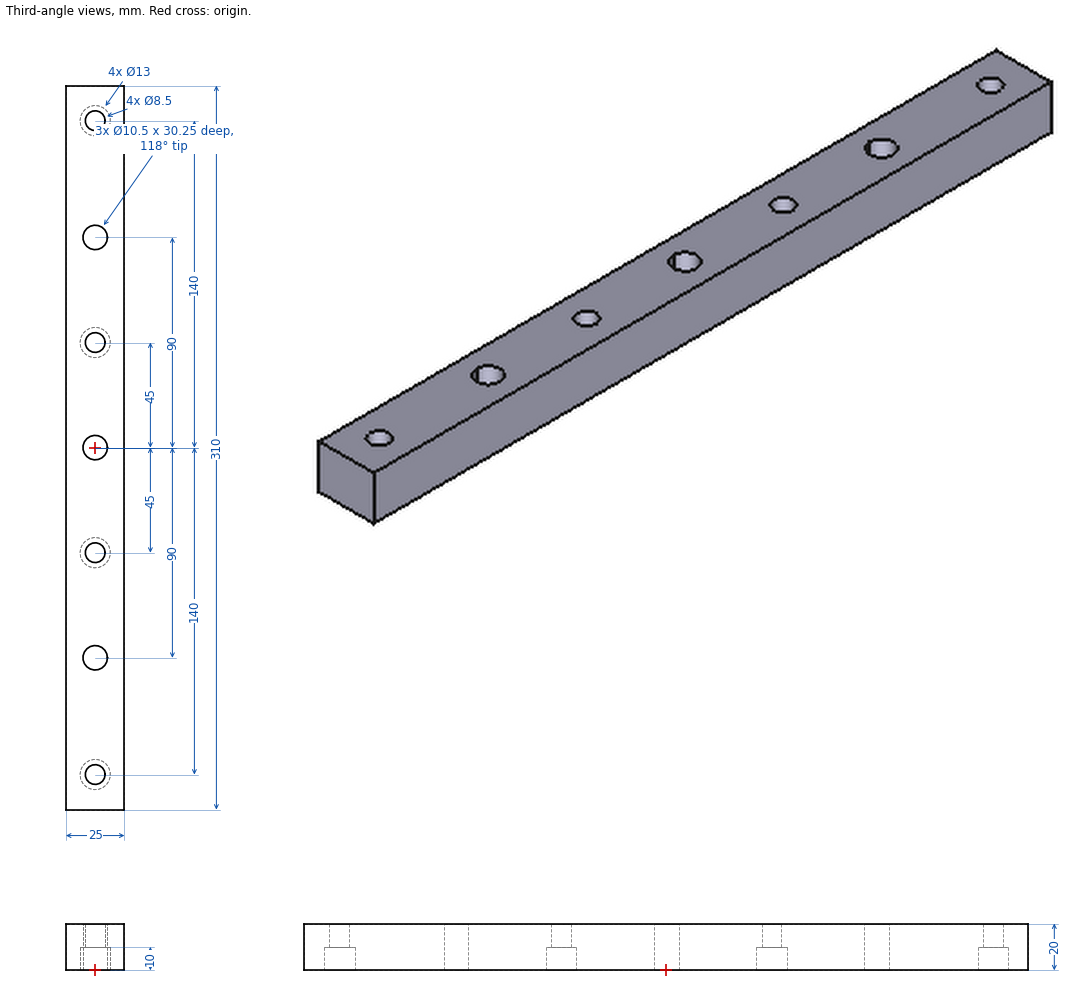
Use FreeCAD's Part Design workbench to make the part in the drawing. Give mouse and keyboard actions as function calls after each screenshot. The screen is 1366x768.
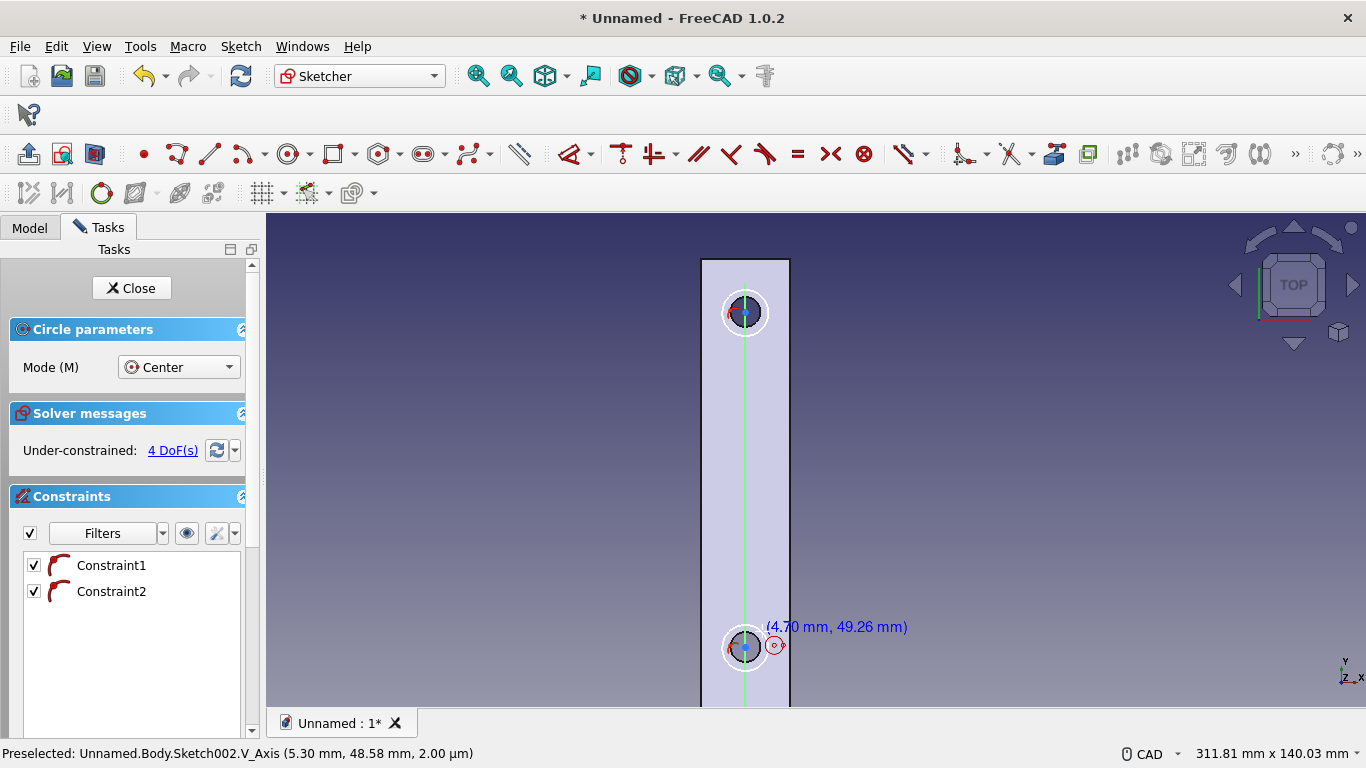
scroll(748, 311, down, 6)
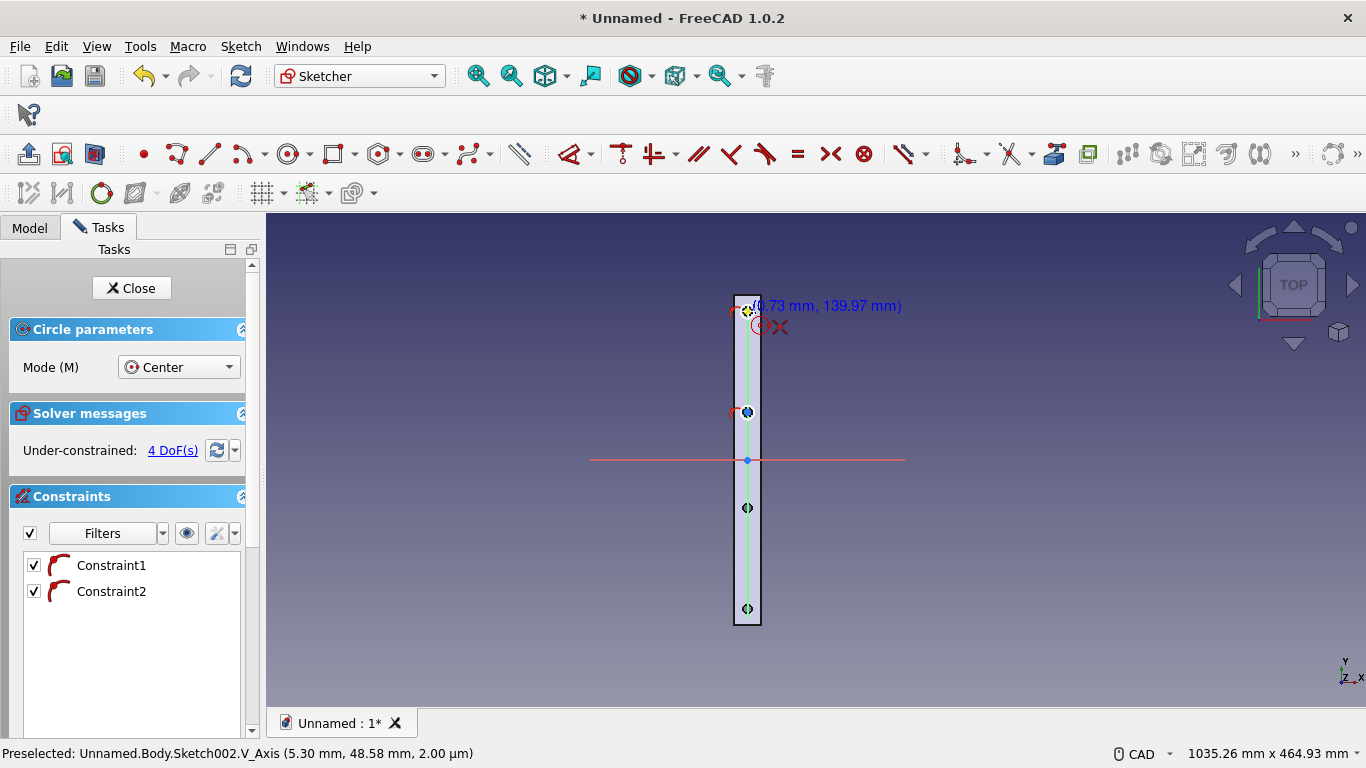
scroll(748, 508, up, 6)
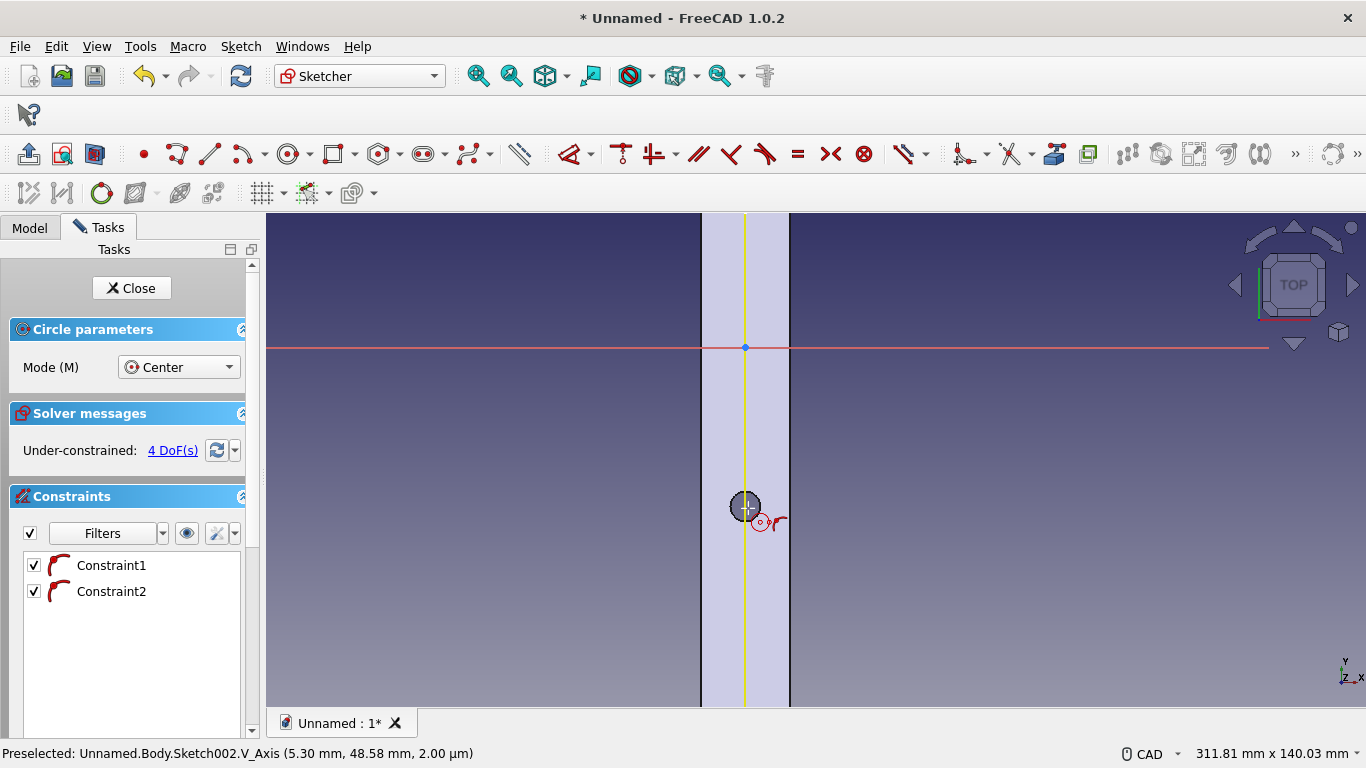
click(745, 507)
click(762, 490)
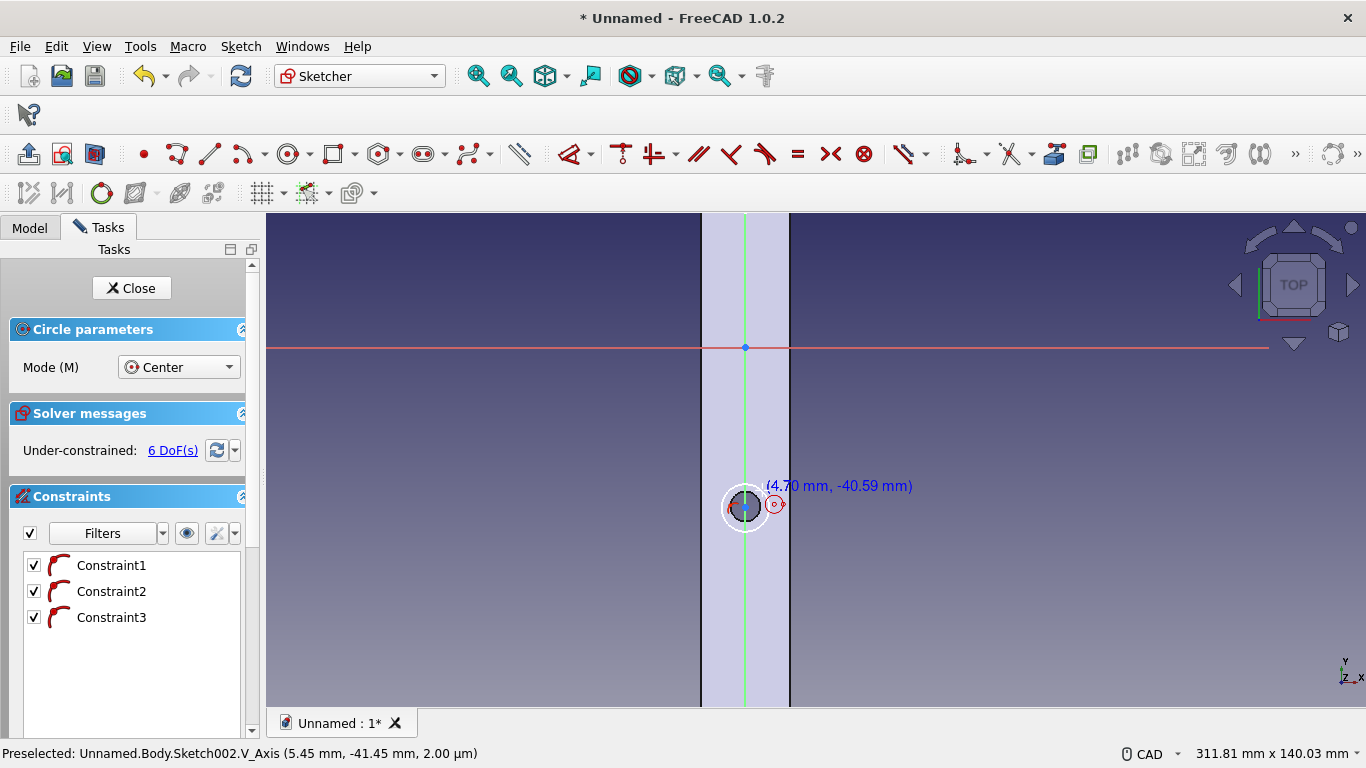
scroll(748, 508, down, 6)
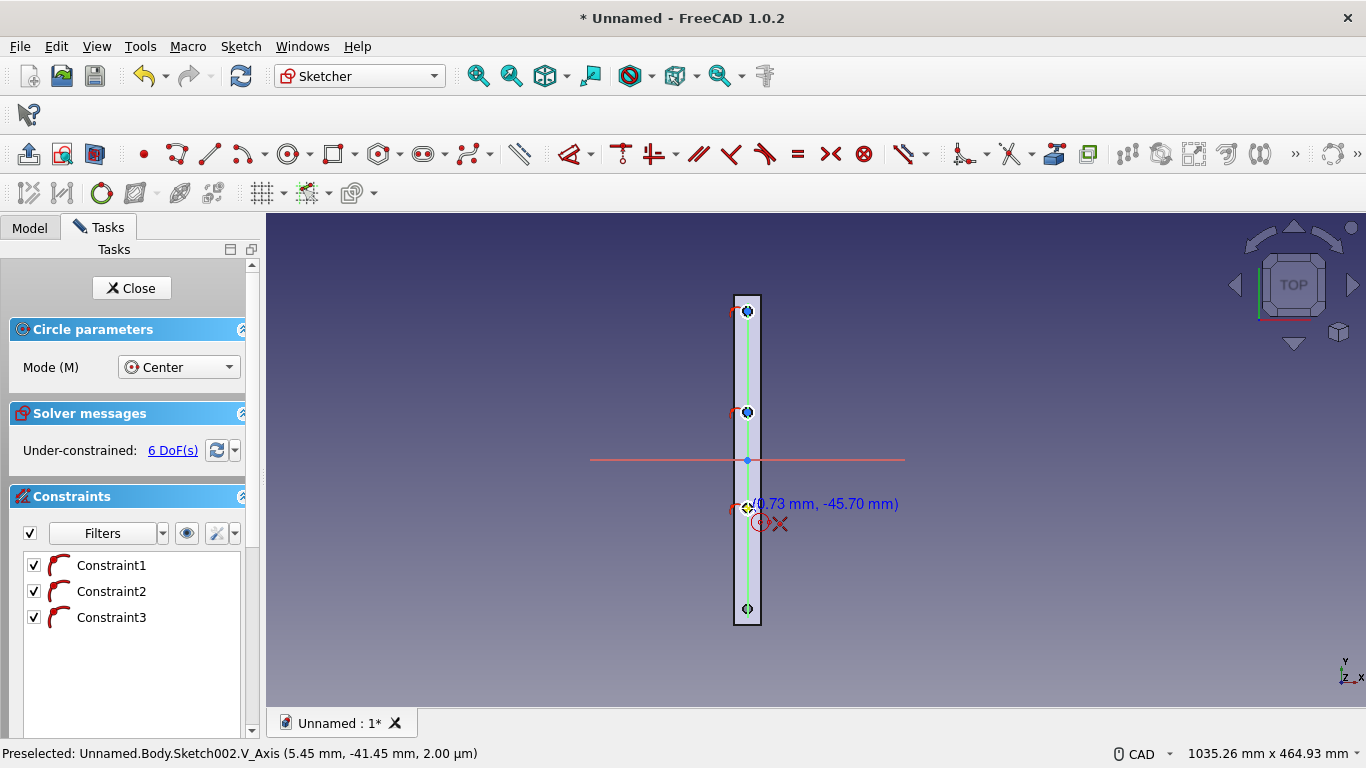
scroll(748, 609, up, 6)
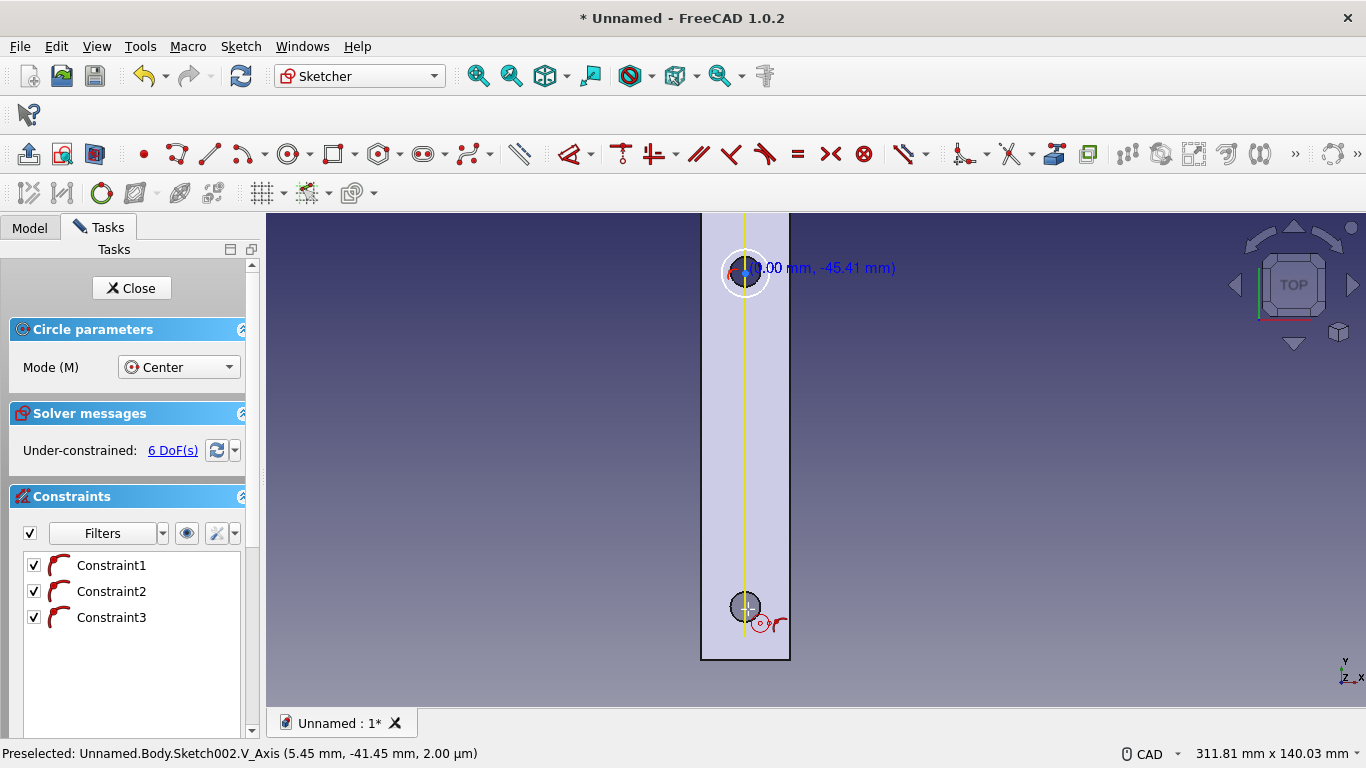
click(745, 607)
click(762, 591)
key(Escape)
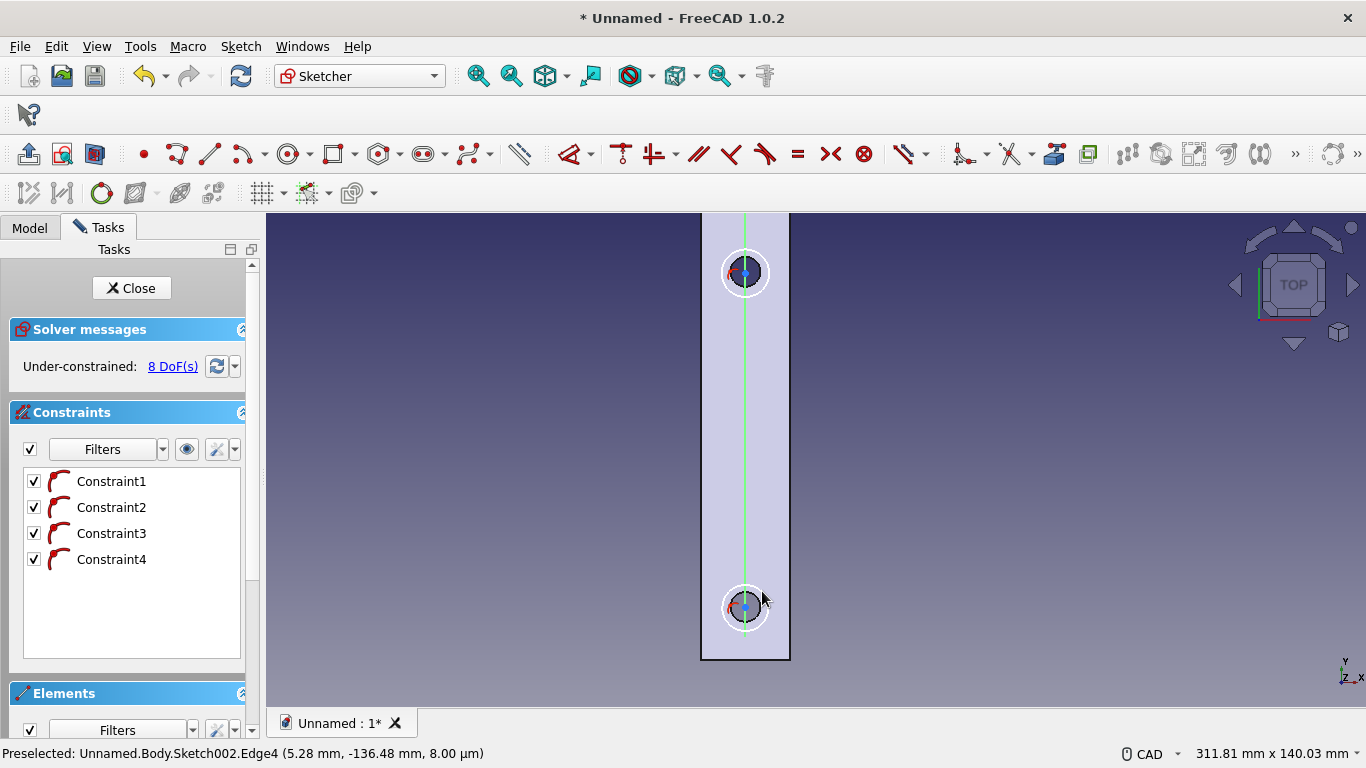
scroll(748, 610, down, 6)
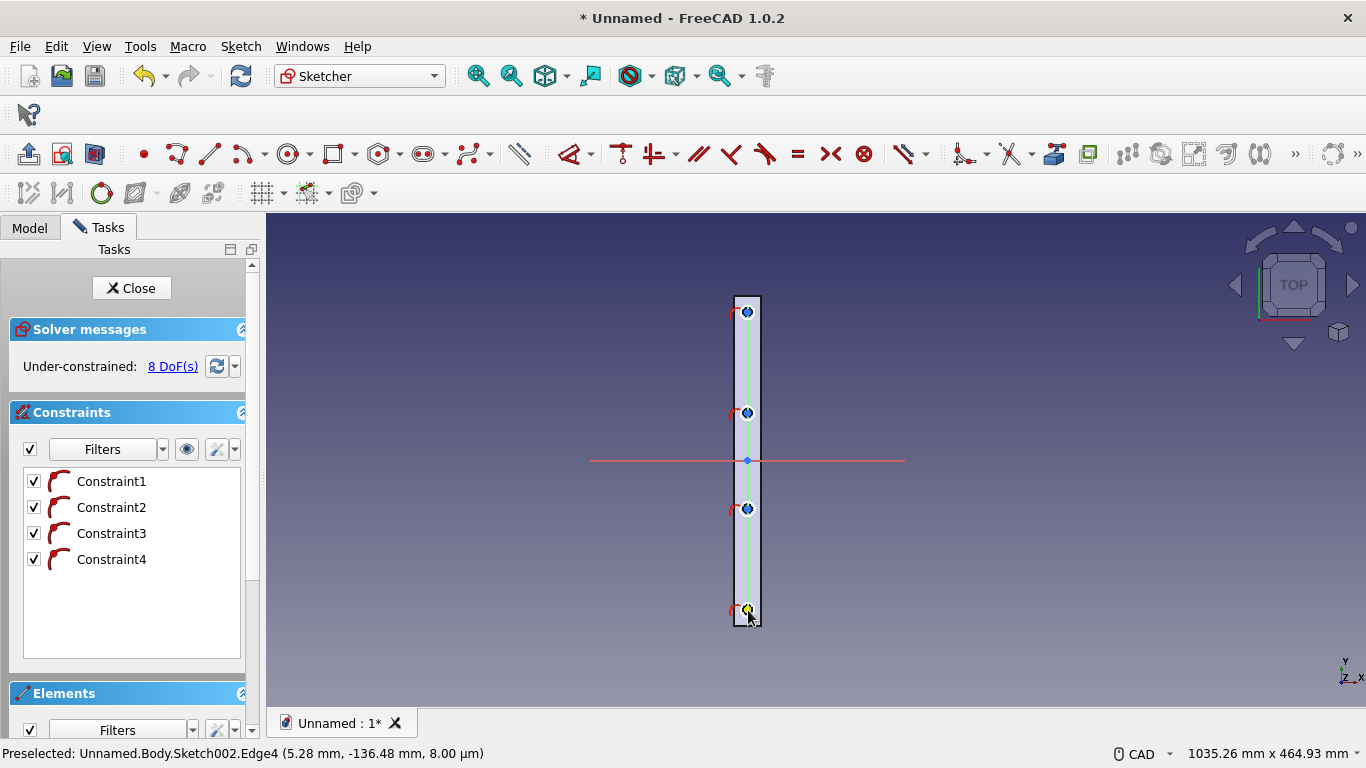
scroll(752, 308, up, 6)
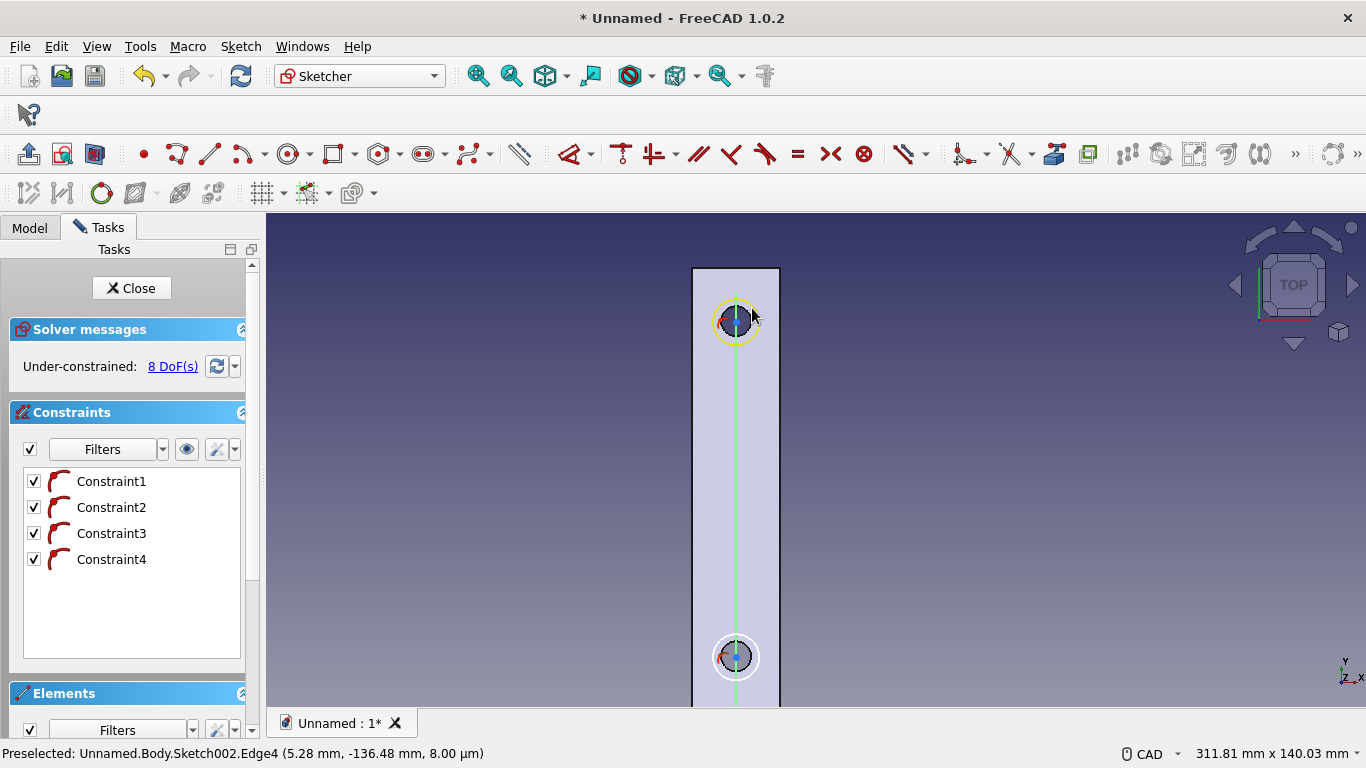
click(752, 306)